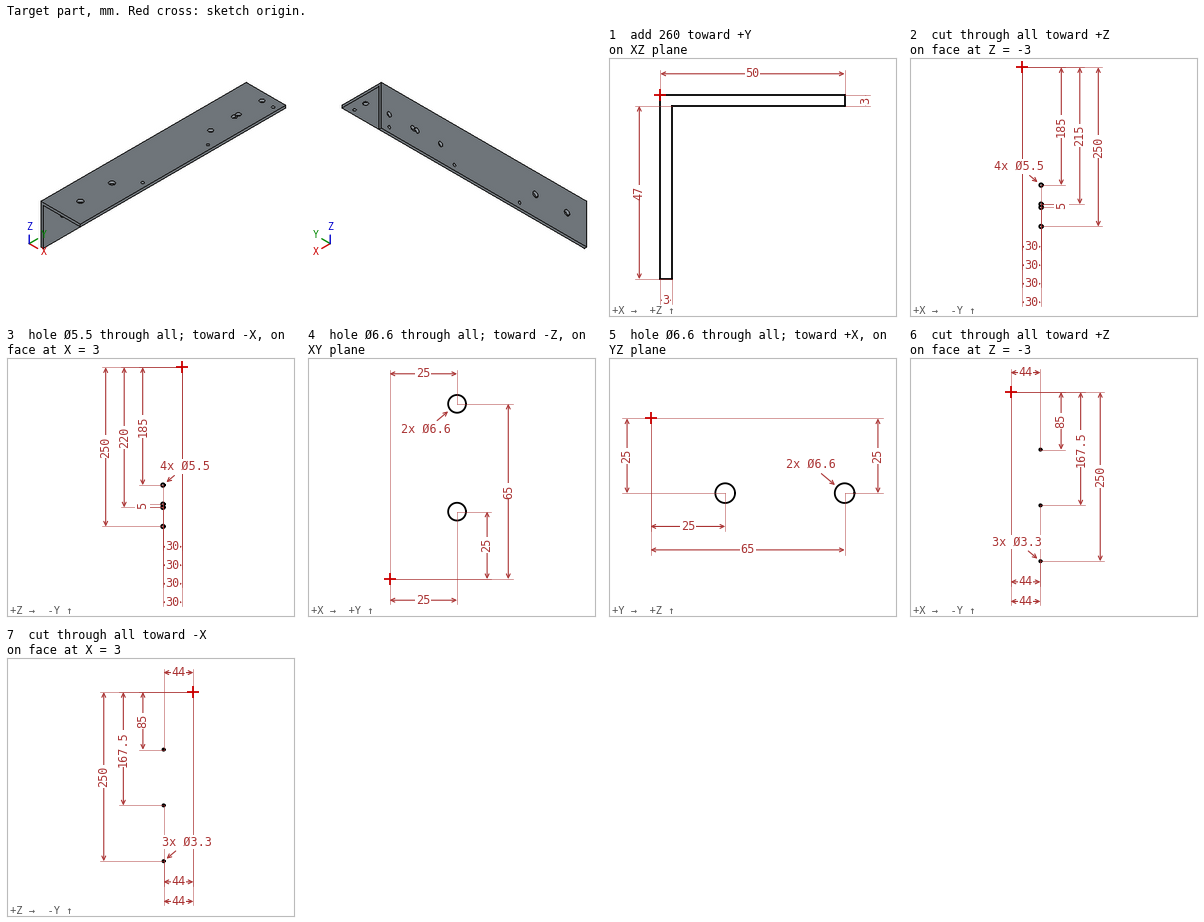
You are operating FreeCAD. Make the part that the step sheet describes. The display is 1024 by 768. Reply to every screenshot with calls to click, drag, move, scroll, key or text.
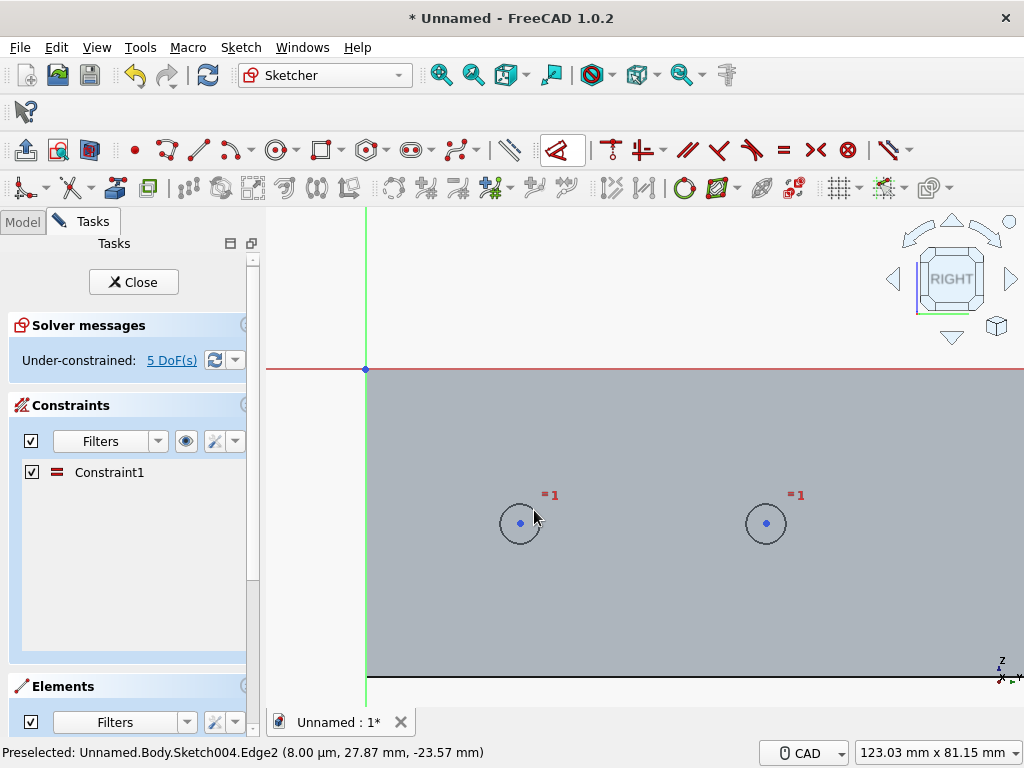
click(780, 510)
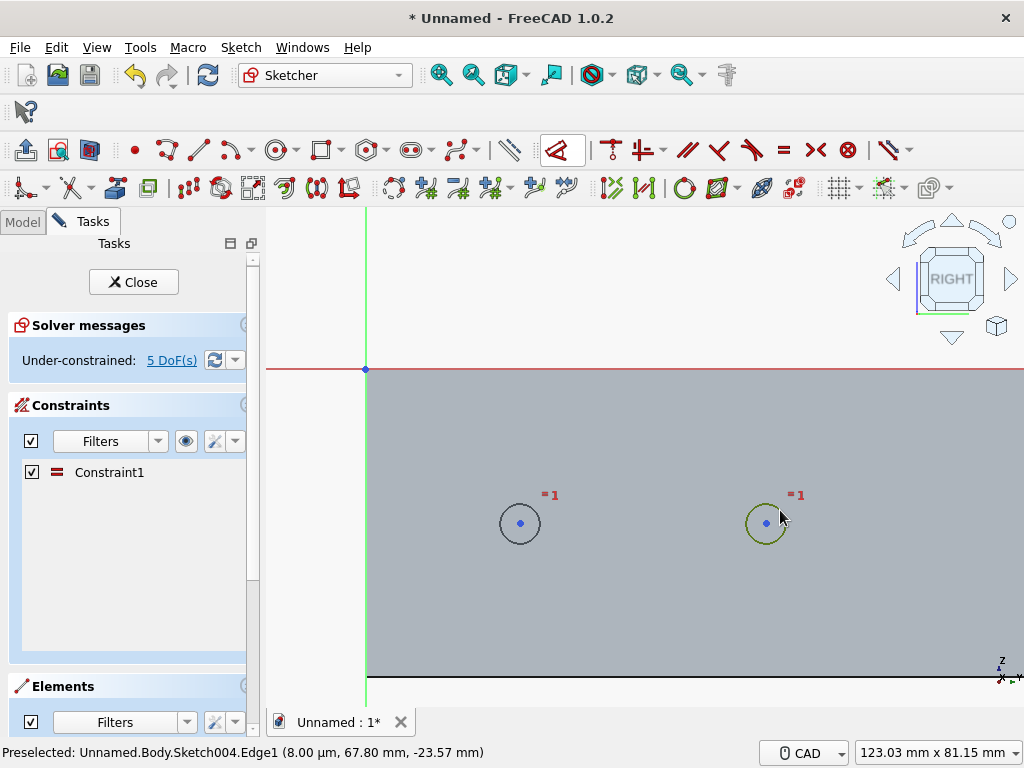
key(k)
key(o)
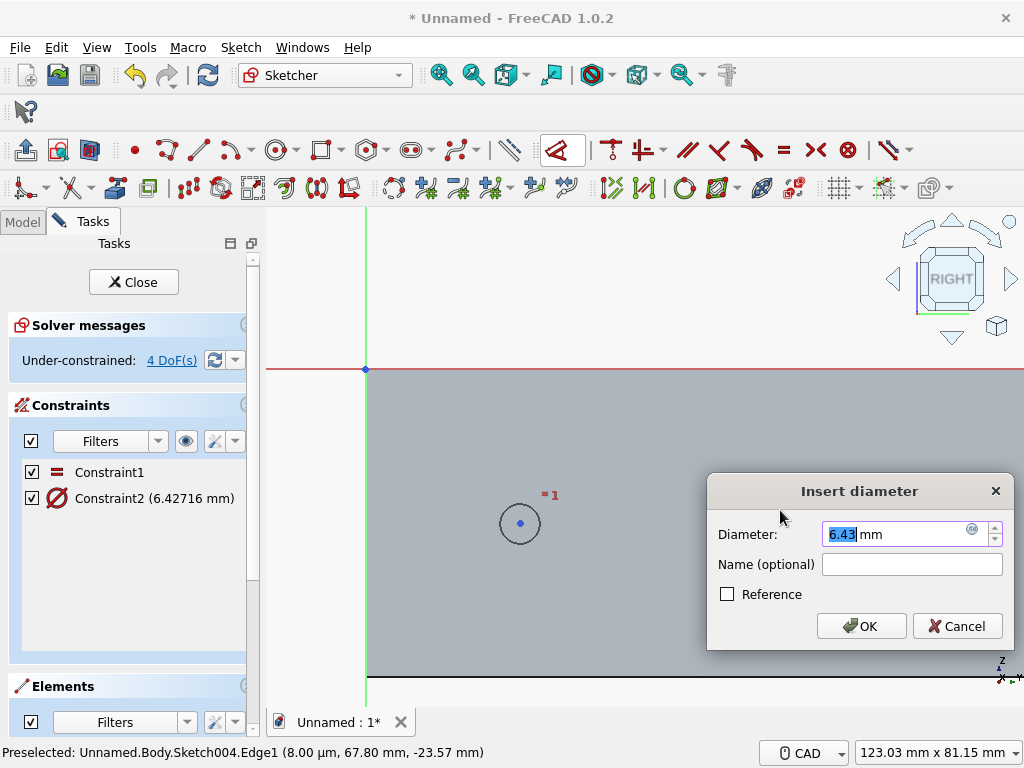
text(6.6)
key(Return)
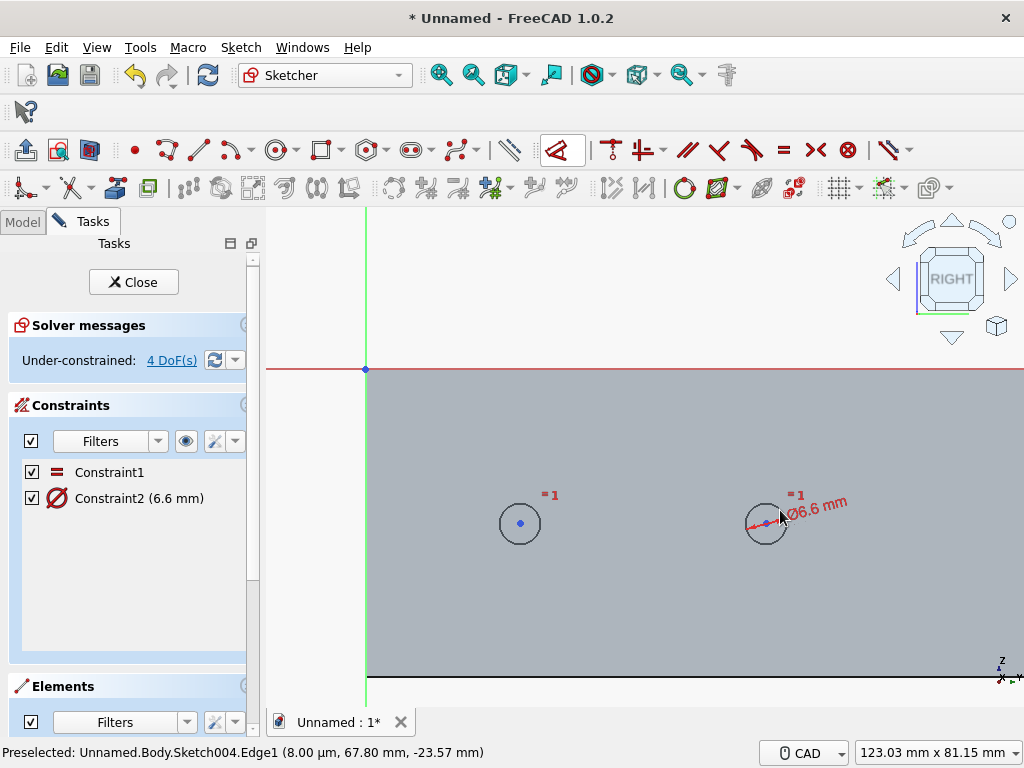
click(766, 524)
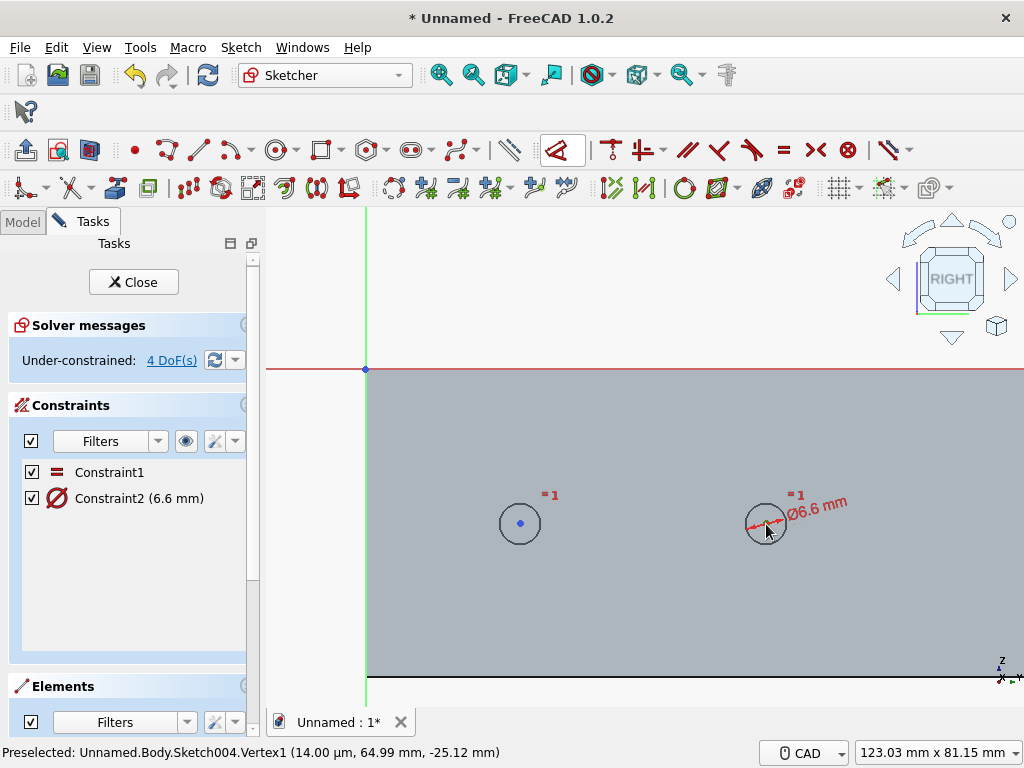
key(l)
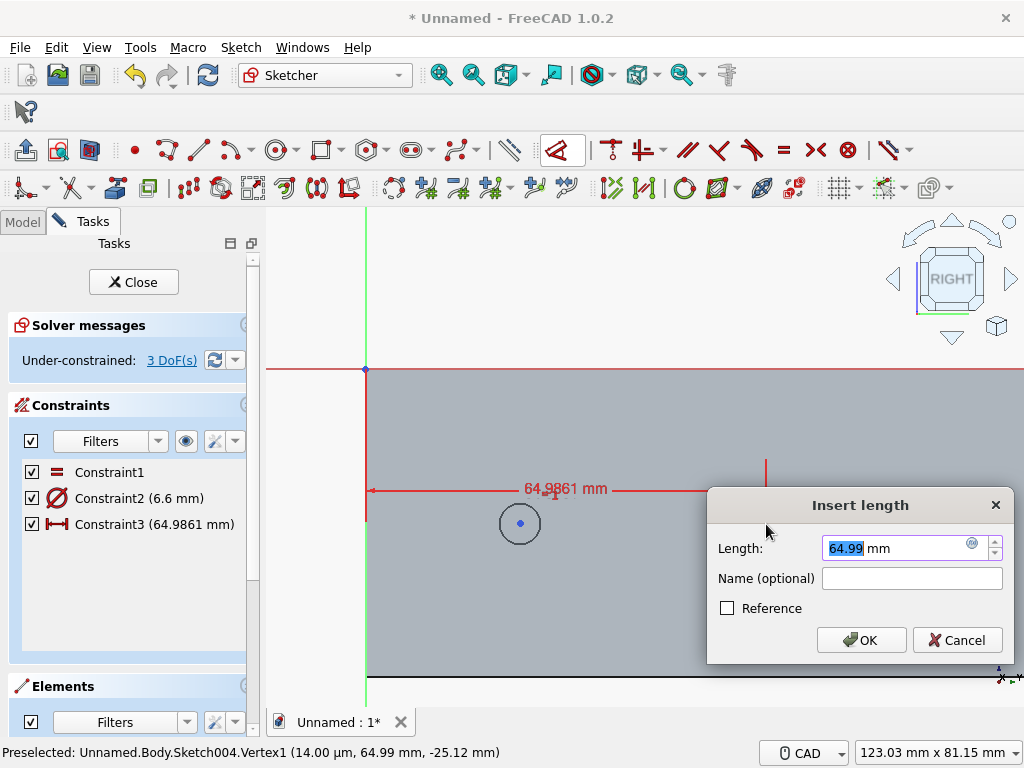
text(65)
key(Return)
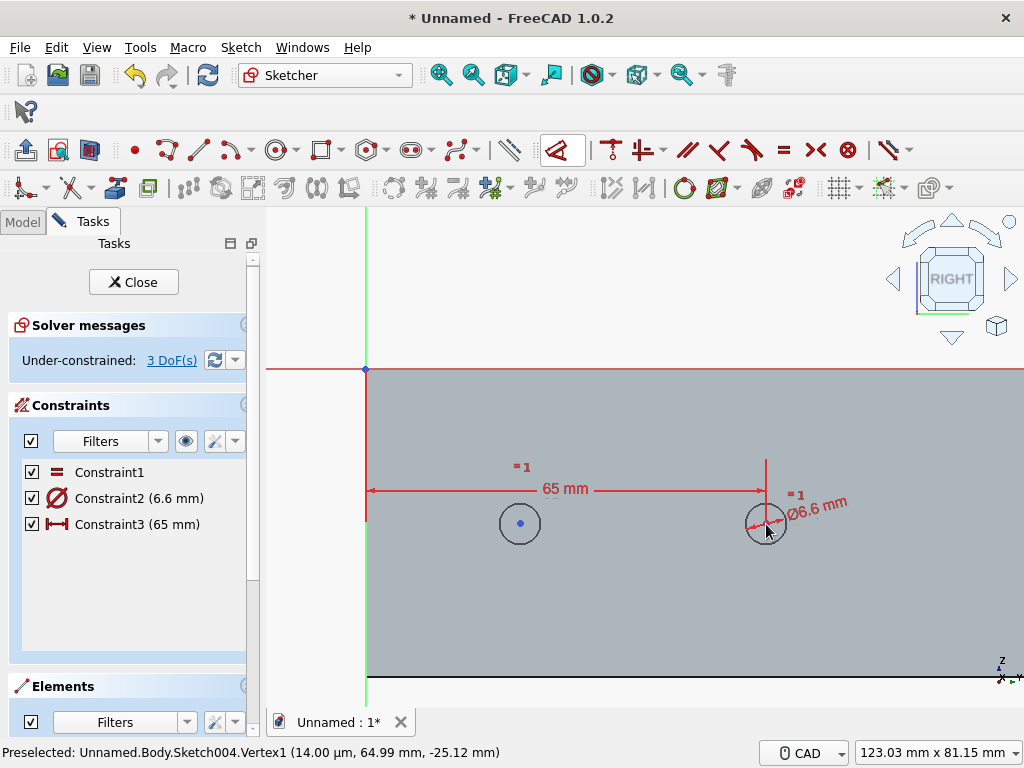
click(766, 524)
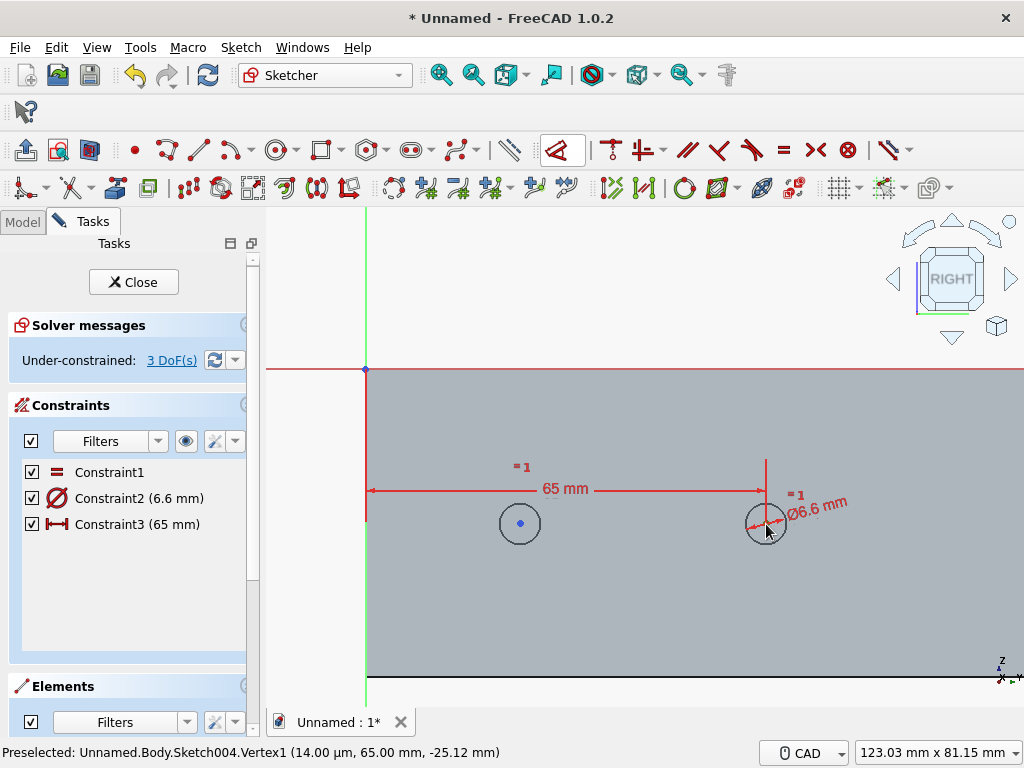
key(i)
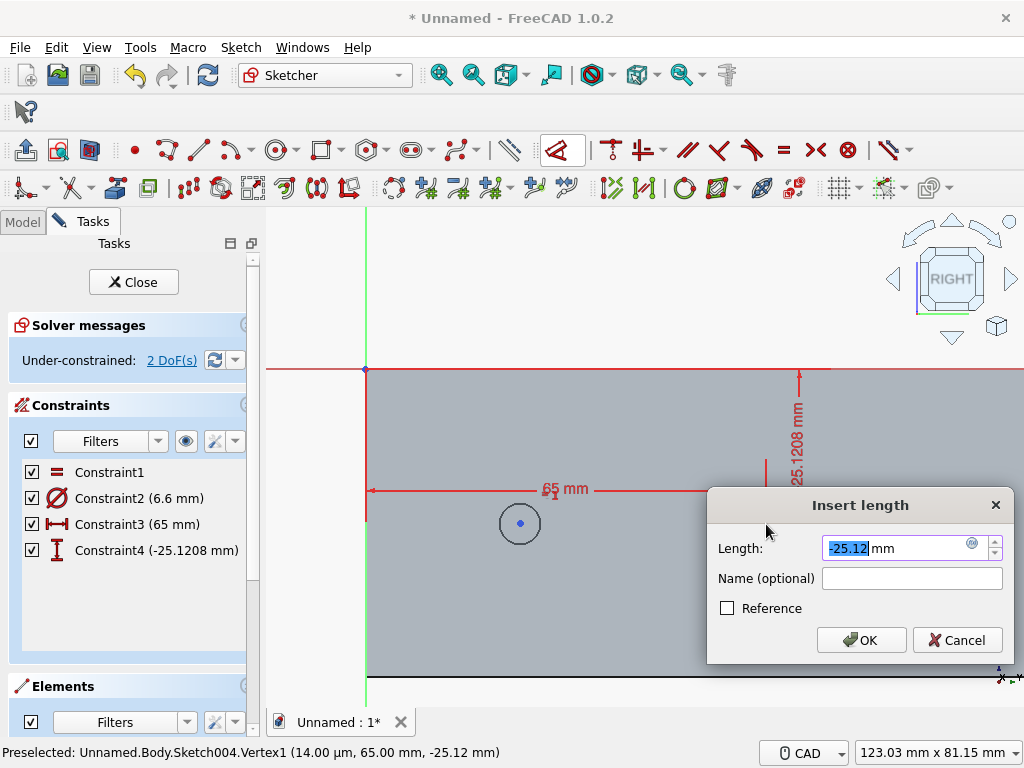
text(-25)
key(Return)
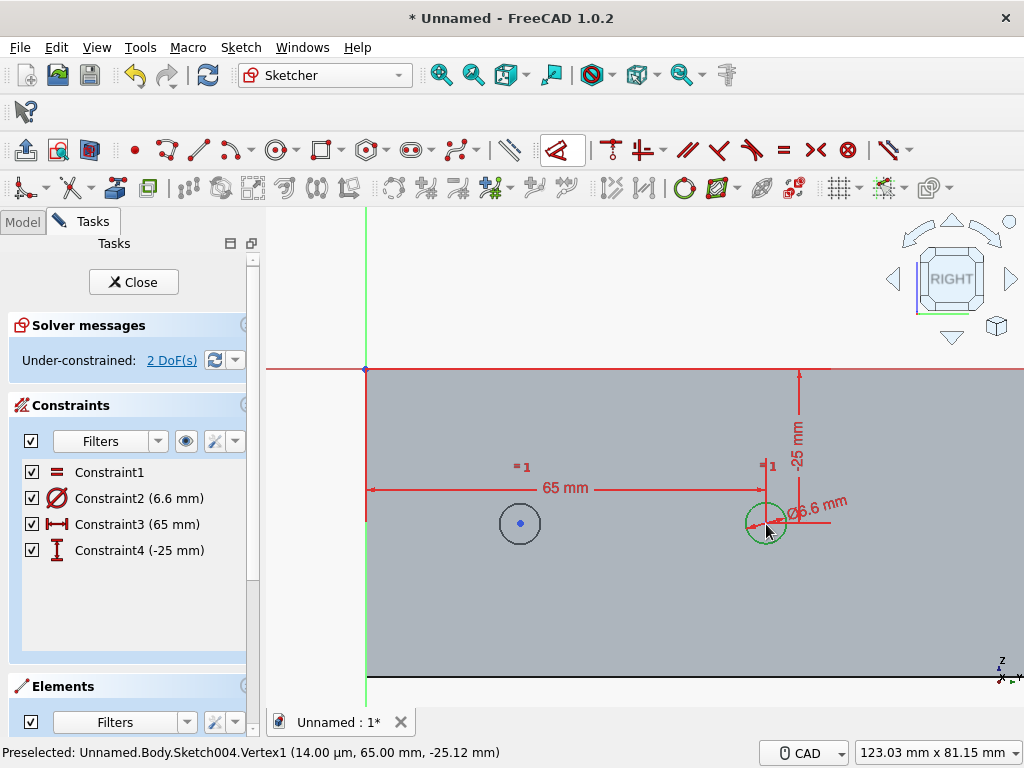
click(520, 524)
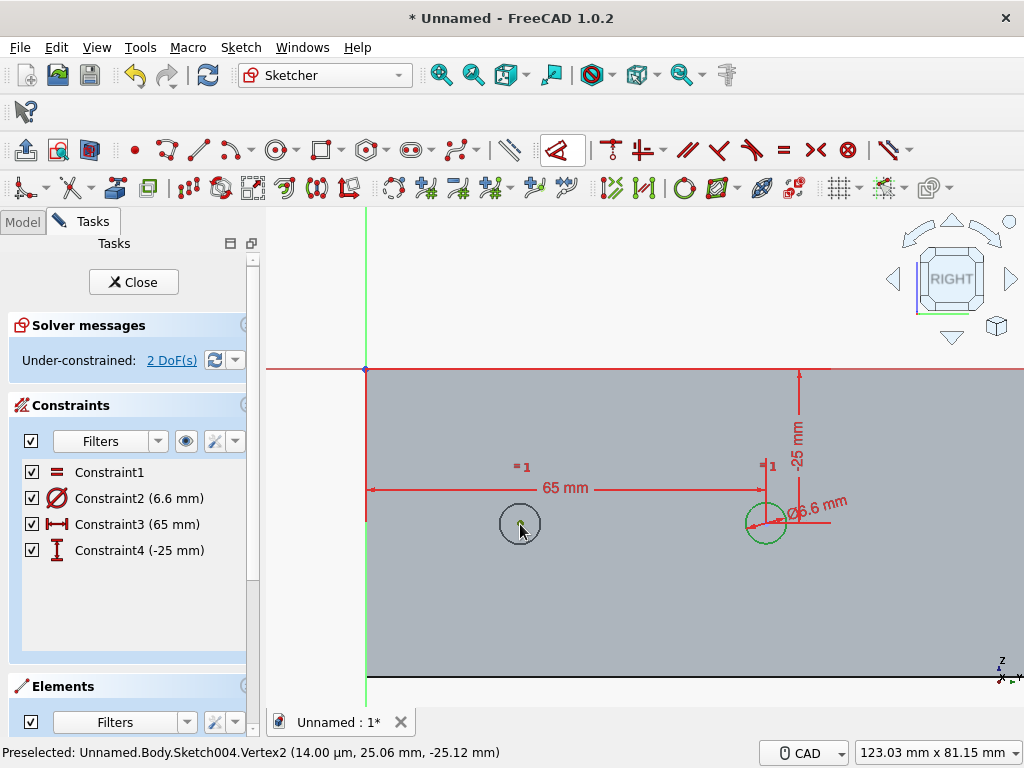
click(580, 150)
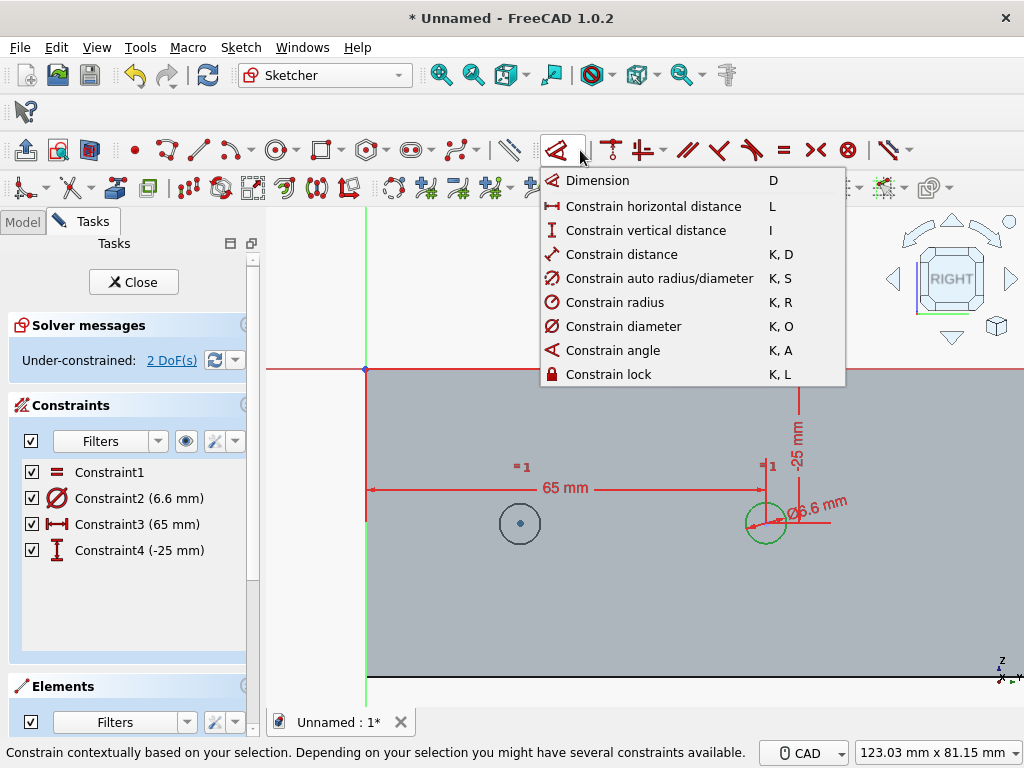
click(693, 206)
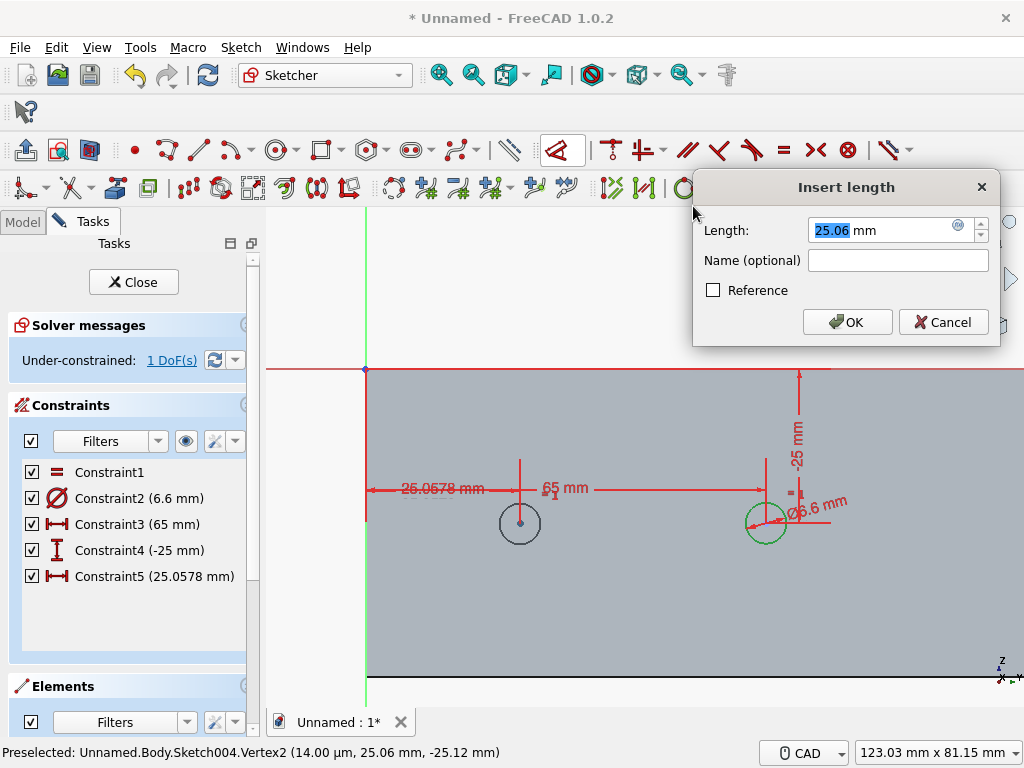
text(25)
key(Return)